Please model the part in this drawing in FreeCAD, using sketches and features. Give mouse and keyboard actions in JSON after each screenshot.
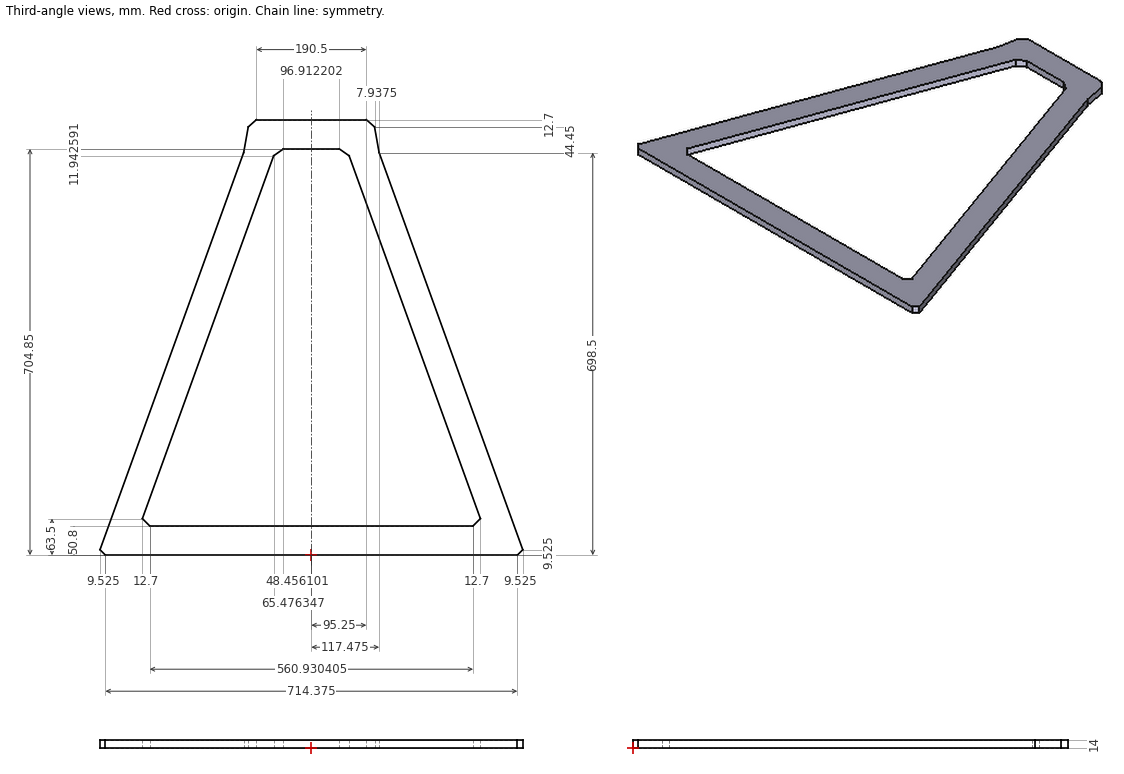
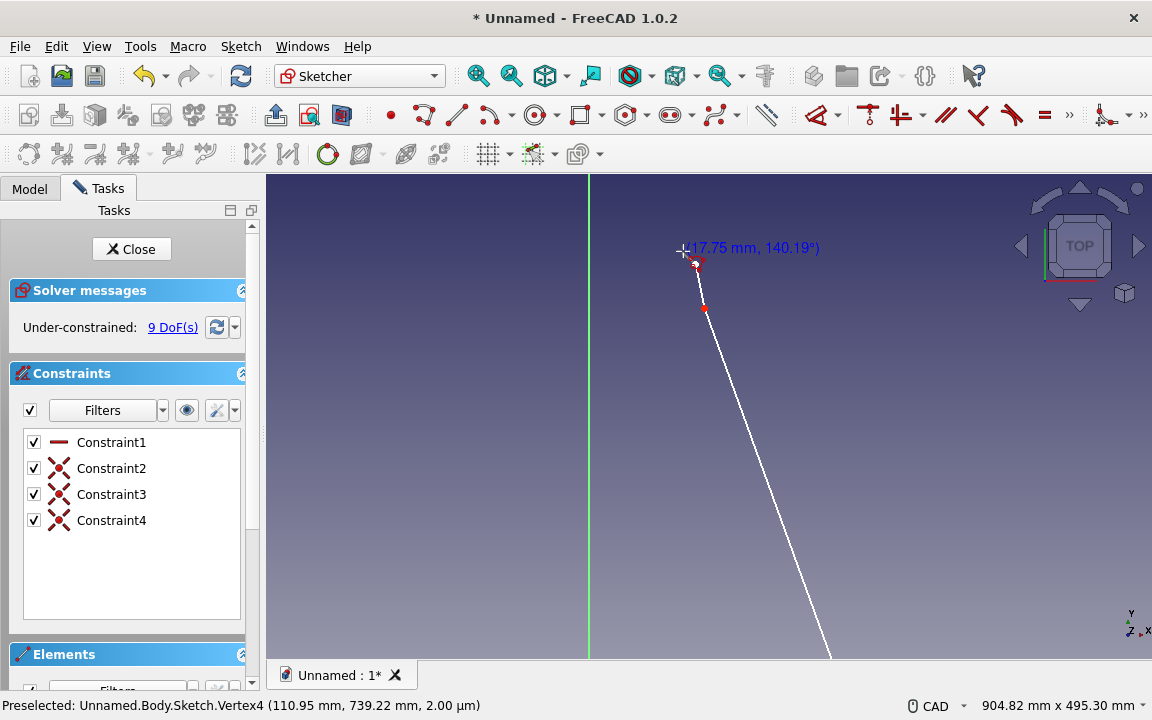
{"action": "left_click", "coordinate": [683, 250]}
{"action": "left_click", "coordinate": [496, 250]}
{"action": "left_click", "coordinate": [482, 263]}
{"action": "left_click", "coordinate": [474, 306]}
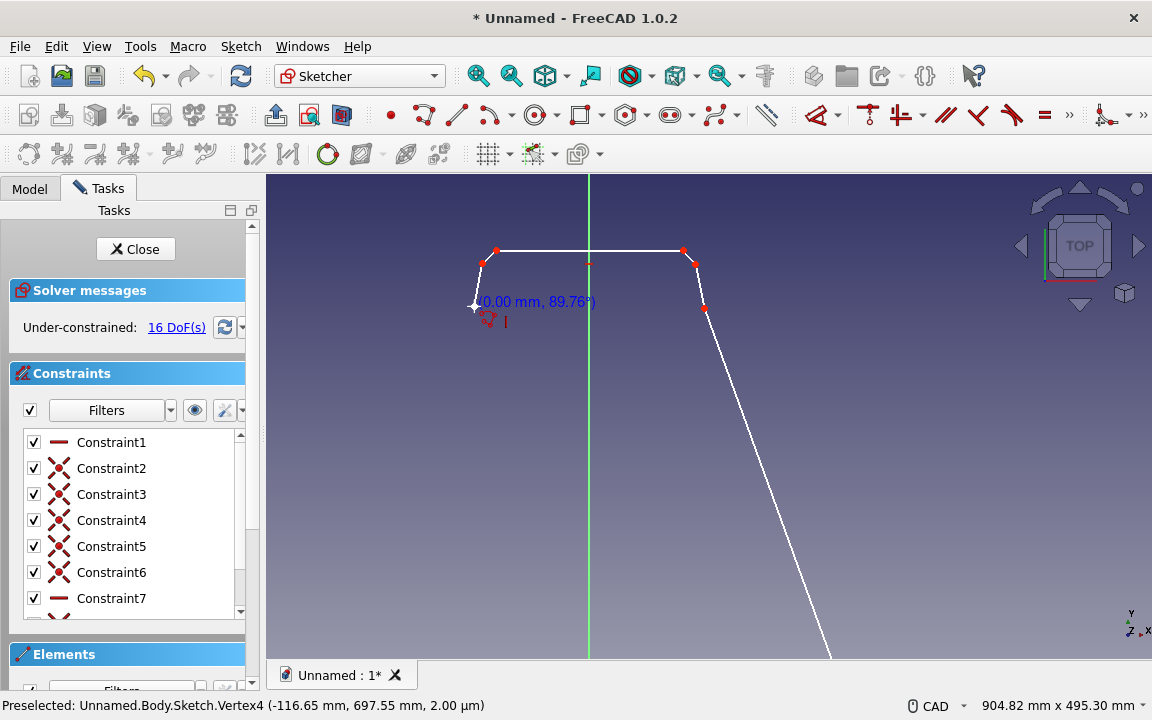
{"action": "scroll", "coordinate": [682, 250], "scroll_direction": "down", "scroll_amount": 4}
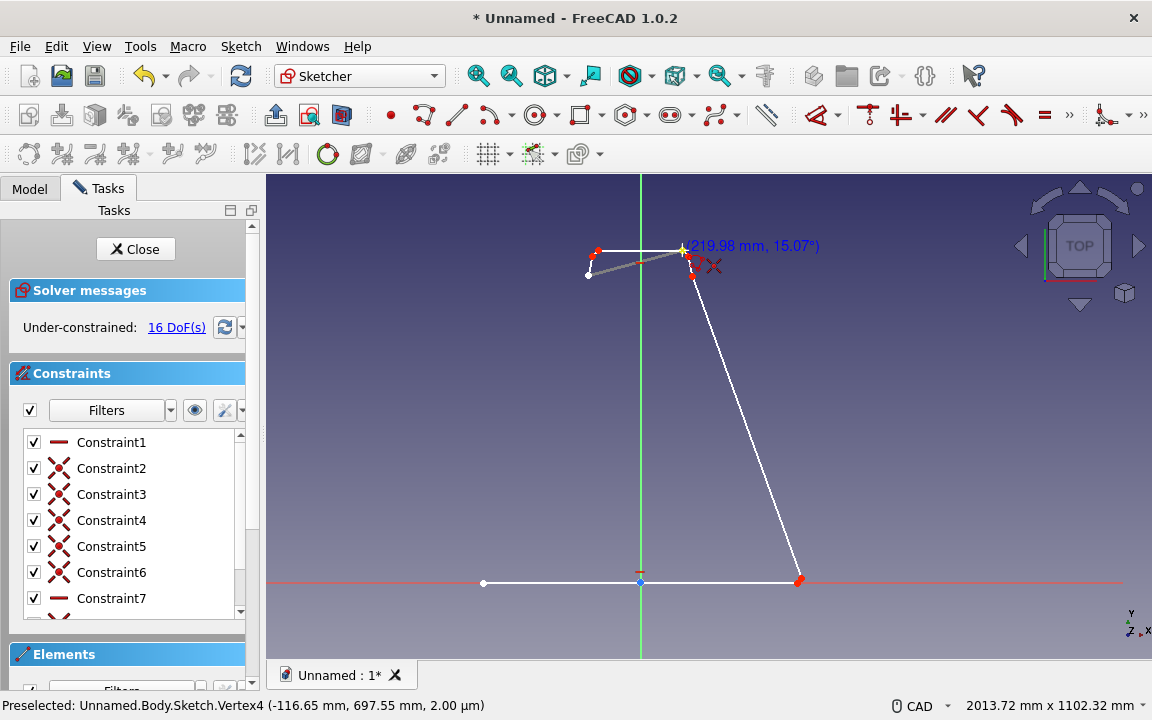
{"action": "scroll", "coordinate": [479, 578], "scroll_direction": "up", "scroll_amount": 7}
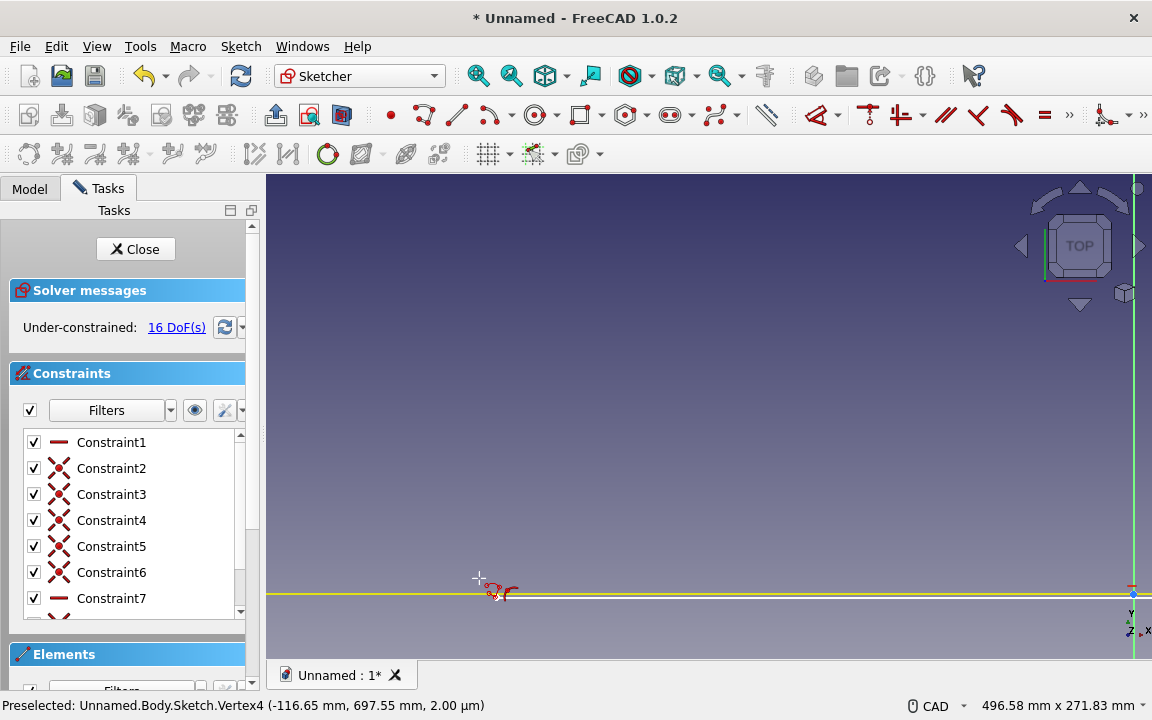
{"action": "left_click", "coordinate": [479, 577]}
{"action": "left_click", "coordinate": [496, 598]}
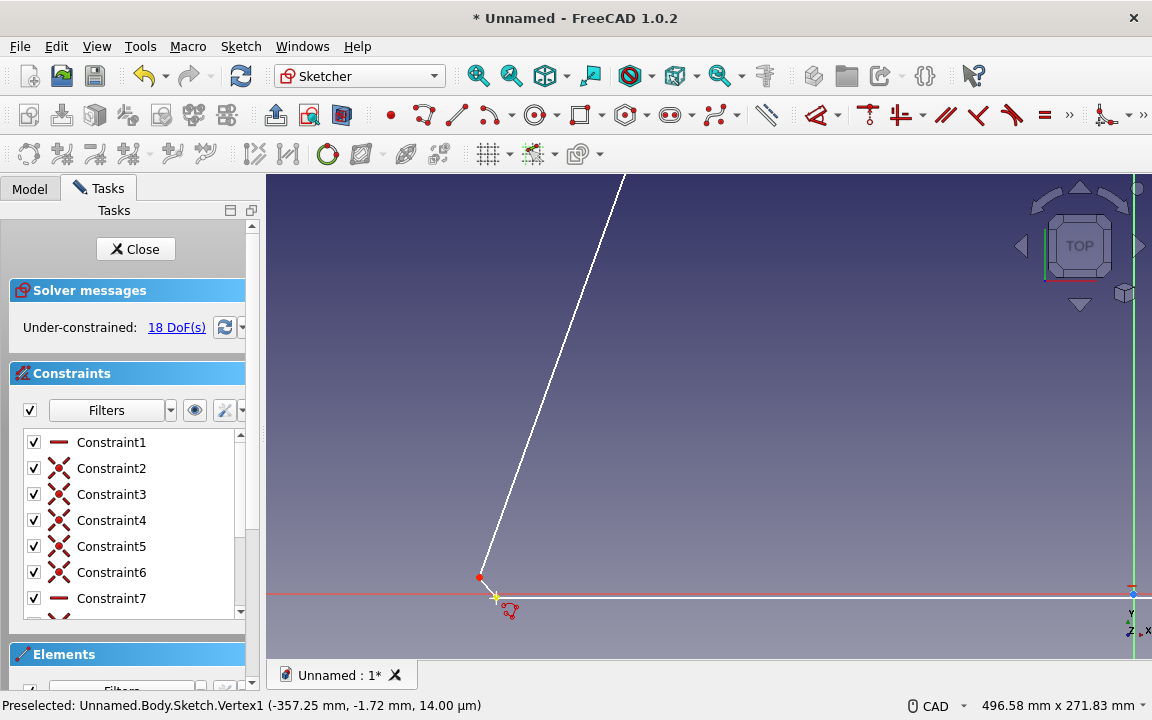
{"action": "scroll", "coordinate": [479, 579], "scroll_direction": "down", "scroll_amount": 7}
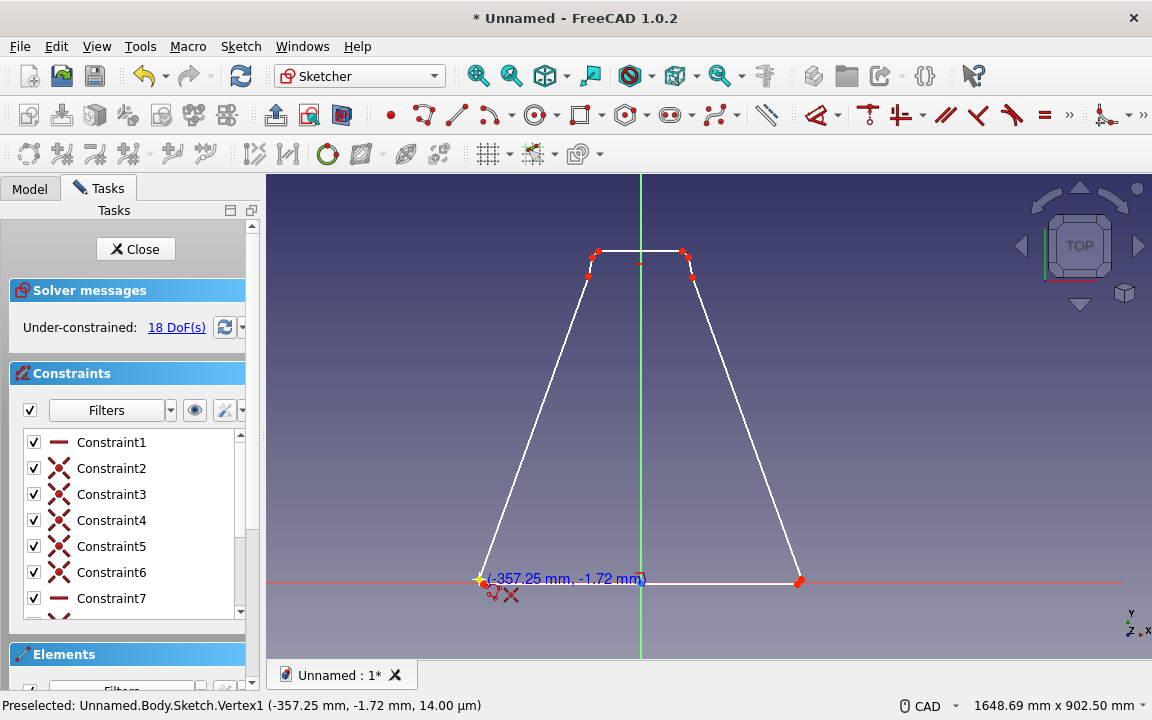
{"action": "left_click", "coordinate": [517, 561]}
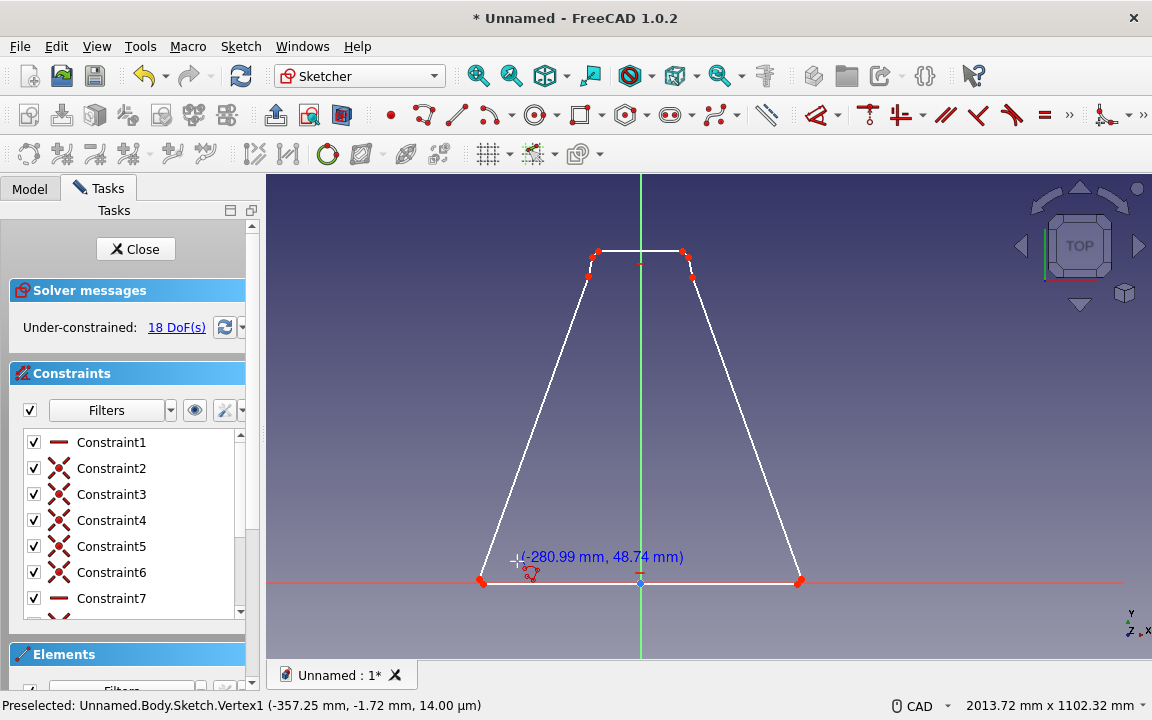
{"action": "scroll", "coordinate": [512, 556], "scroll_direction": "up", "scroll_amount": 4}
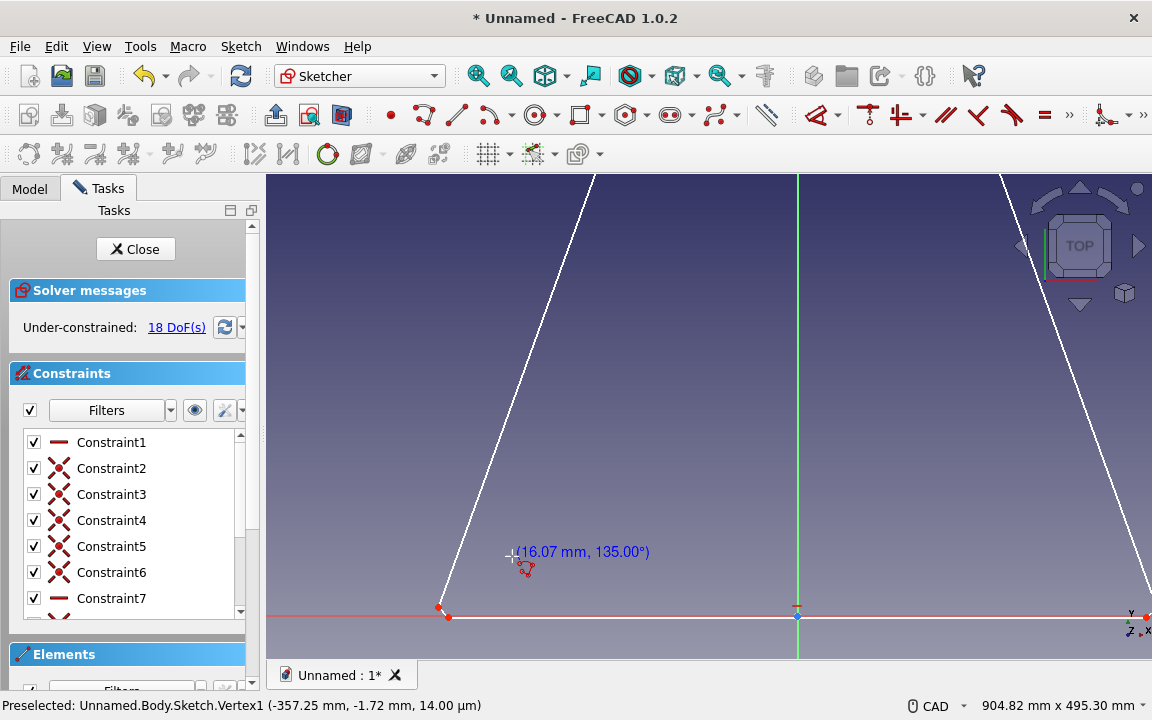
{"action": "left_click", "coordinate": [511, 554]}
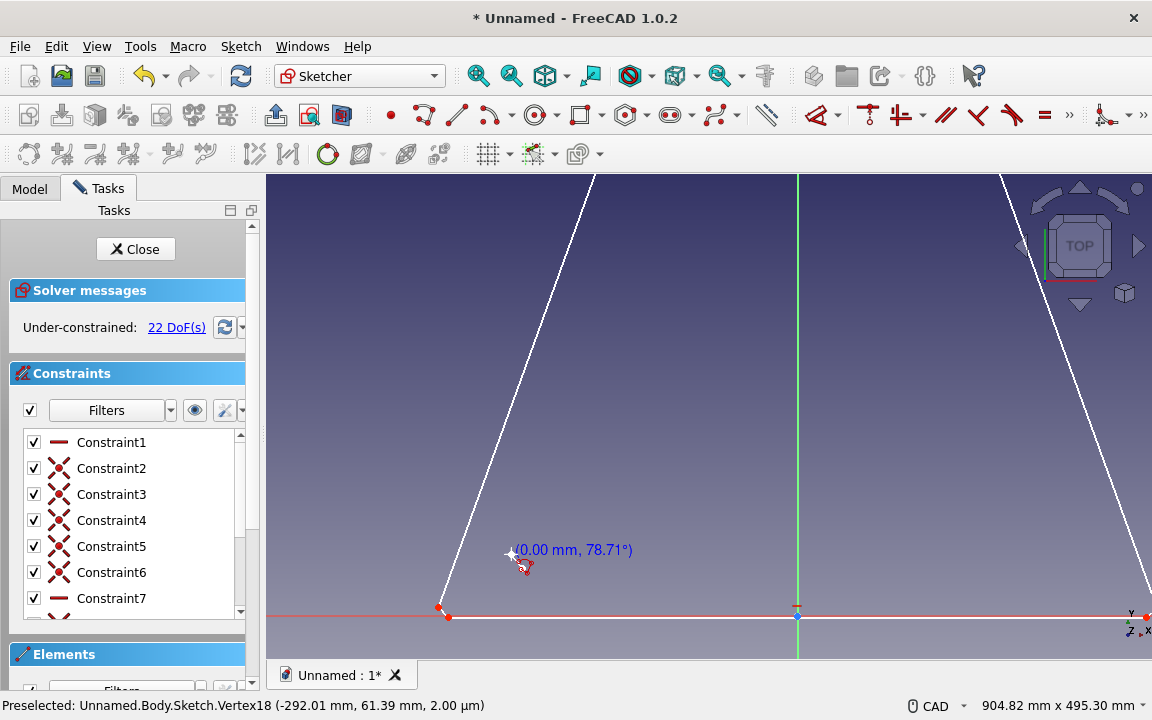
{"action": "scroll", "coordinate": [512, 556], "scroll_direction": "down", "scroll_amount": 4}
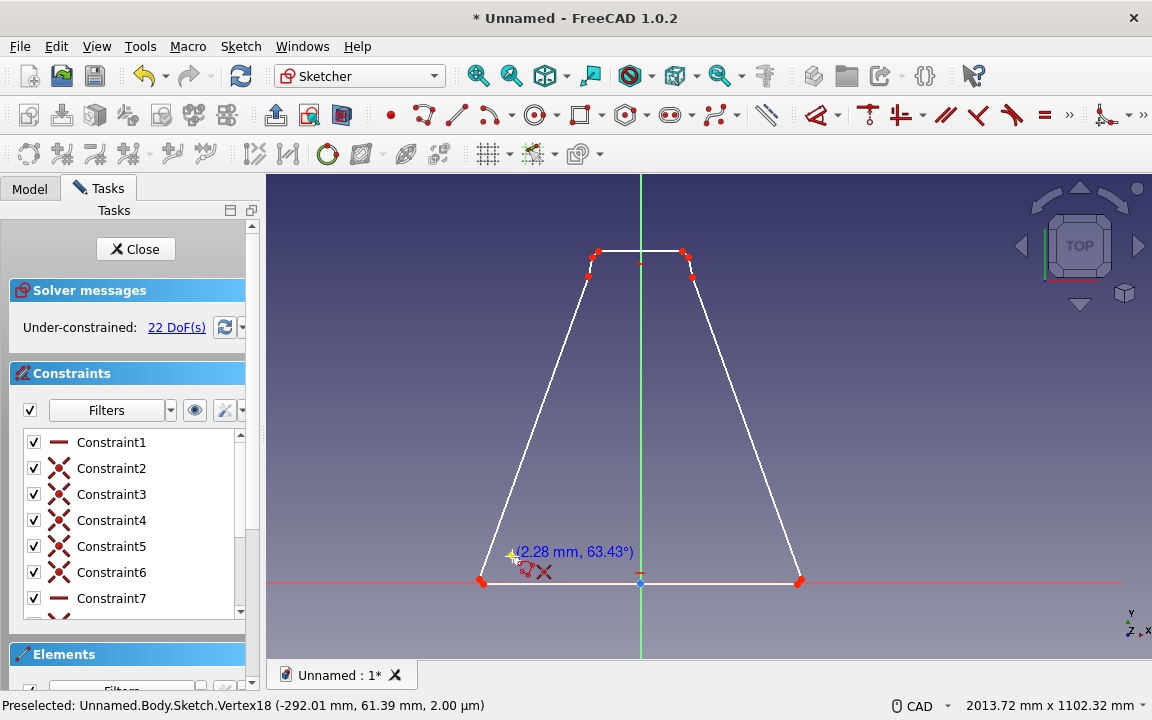
{"action": "left_click", "coordinate": [612, 279]}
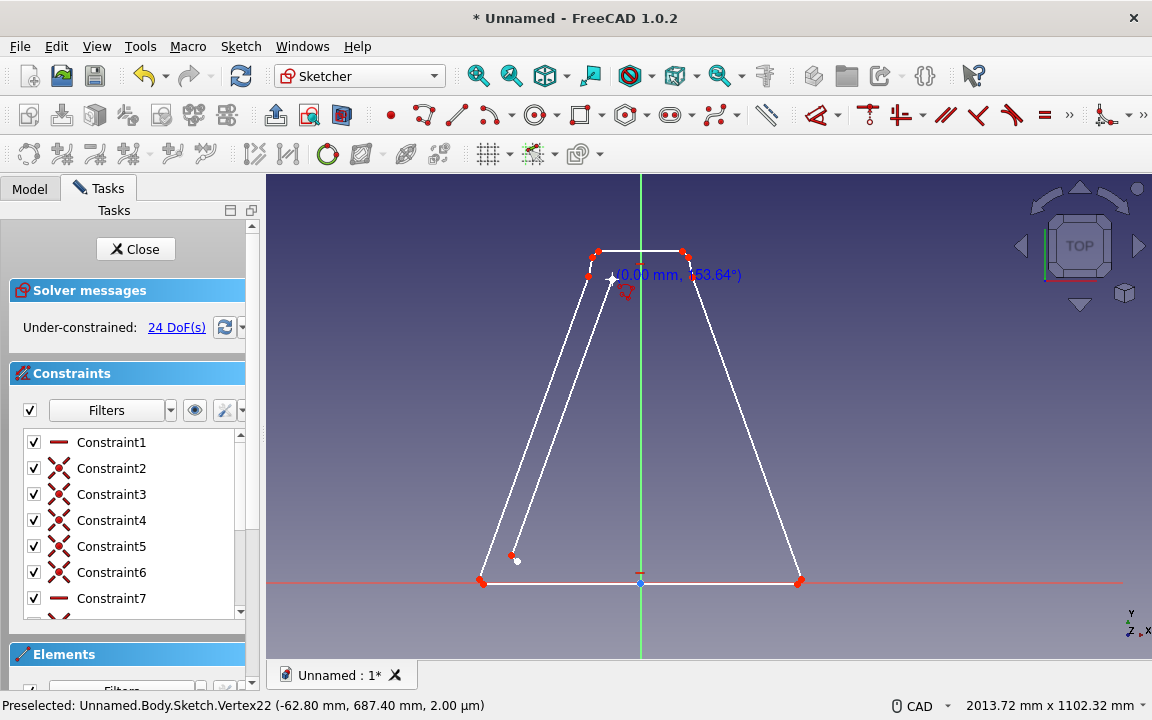
{"action": "scroll", "coordinate": [619, 273], "scroll_direction": "up", "scroll_amount": 3}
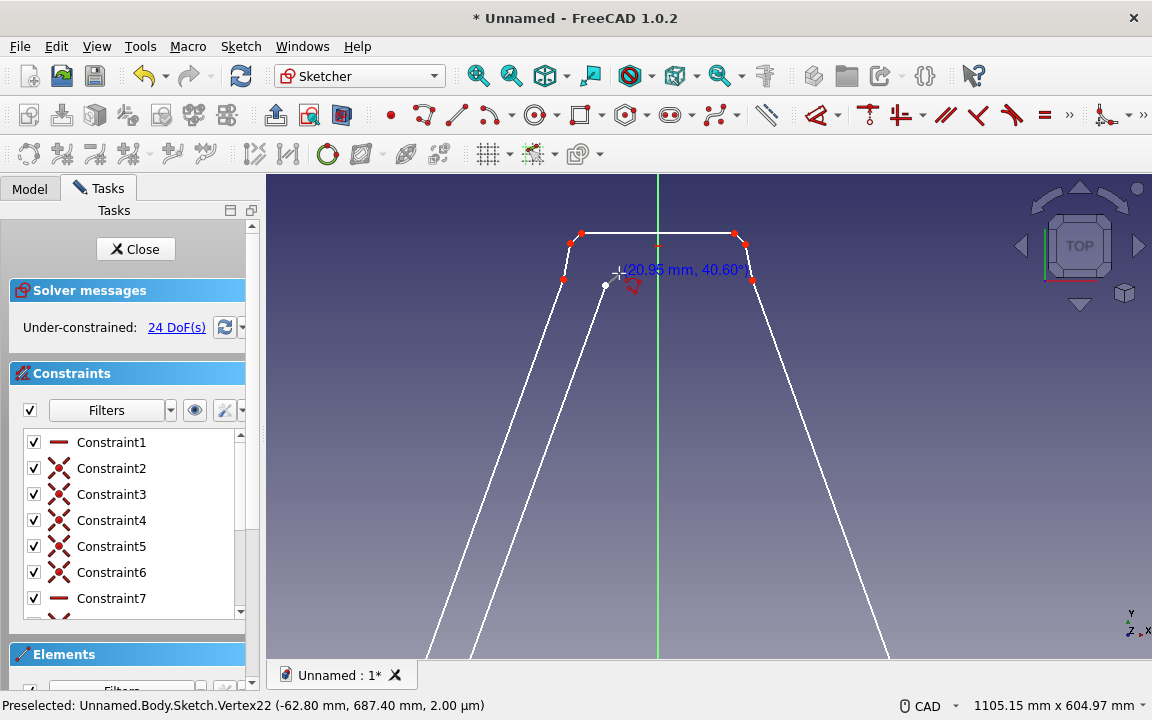
{"action": "left_click", "coordinate": [619, 273]}
{"action": "left_click", "coordinate": [697, 273]}
{"action": "left_click", "coordinate": [711, 283]}